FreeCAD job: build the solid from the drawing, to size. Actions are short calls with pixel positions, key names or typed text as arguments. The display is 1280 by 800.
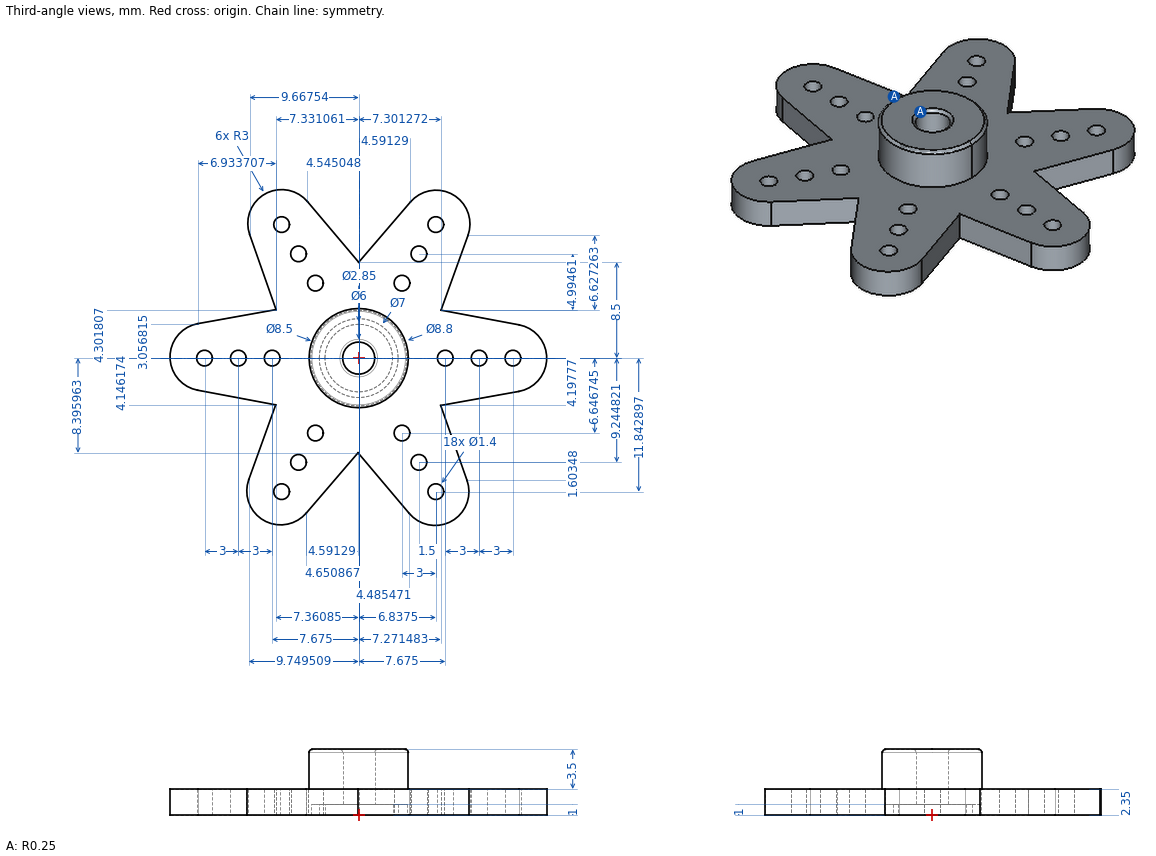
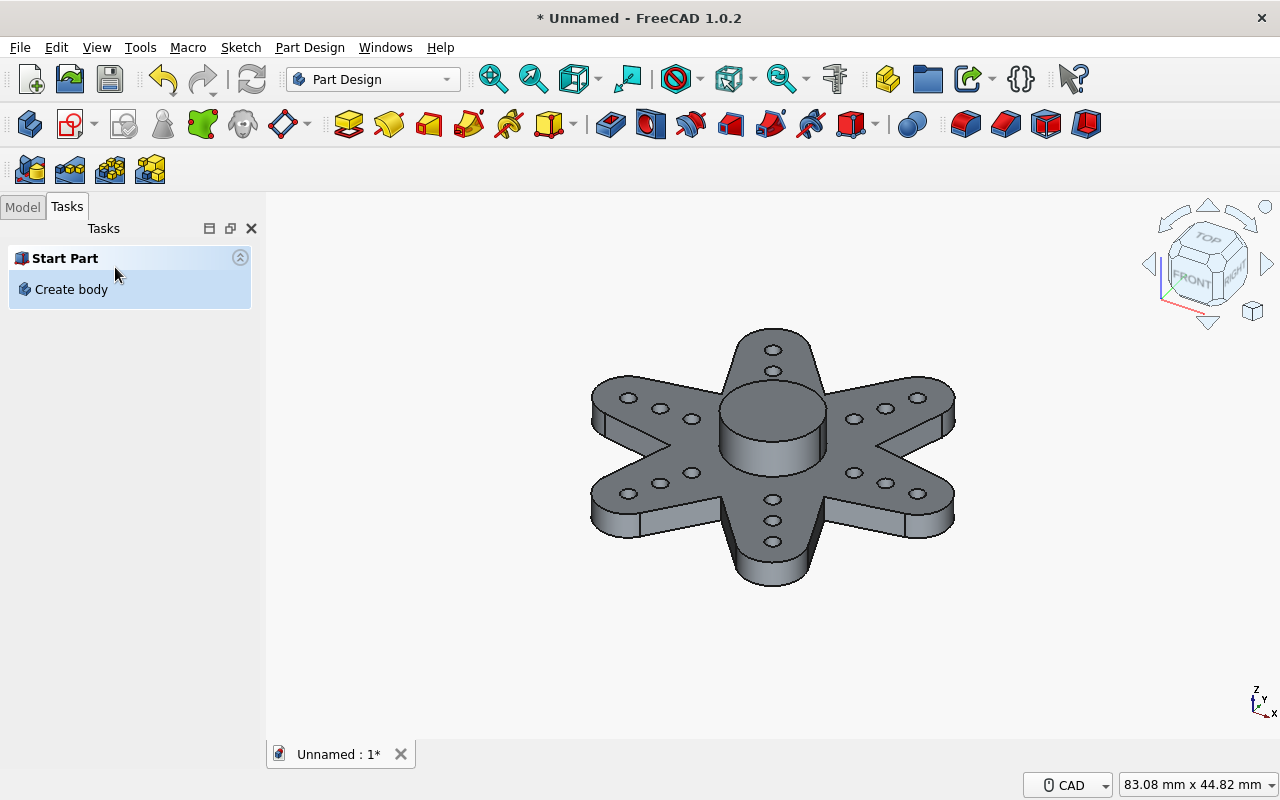
click(773, 410)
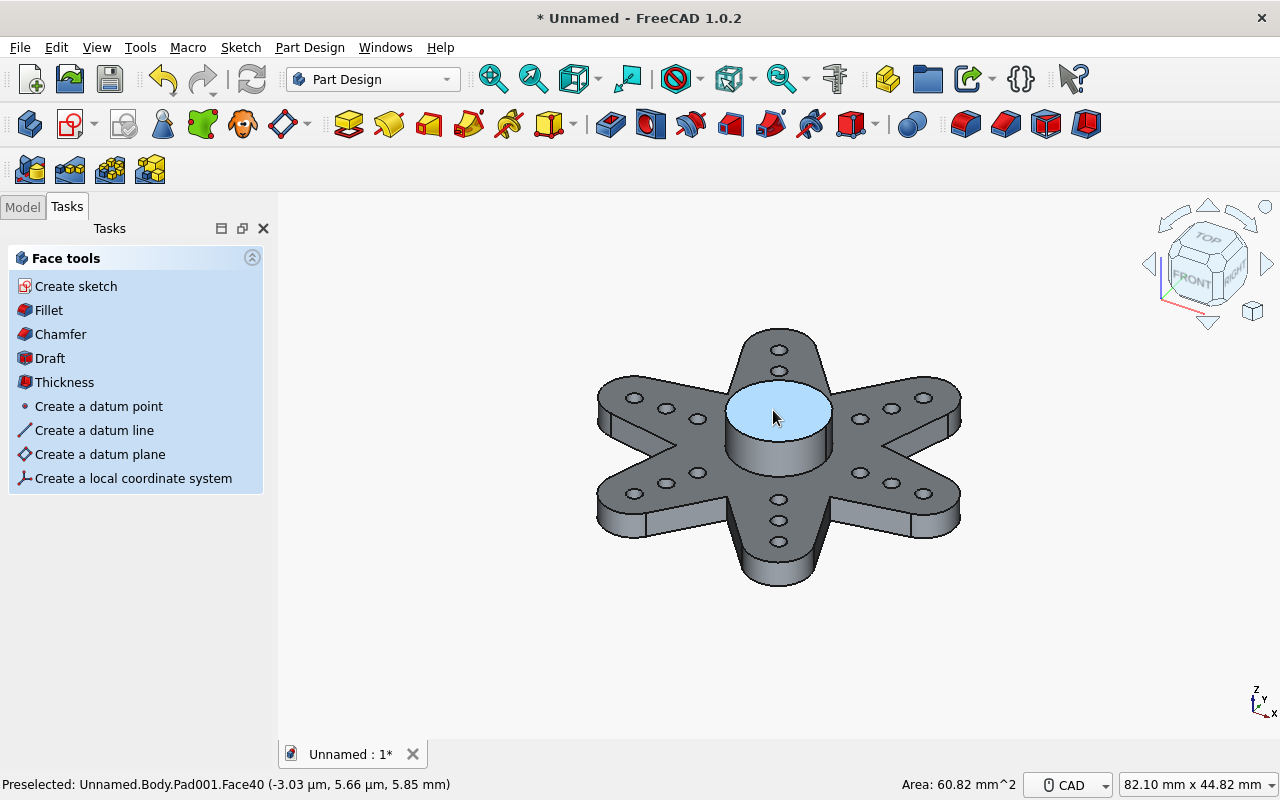
click(70, 124)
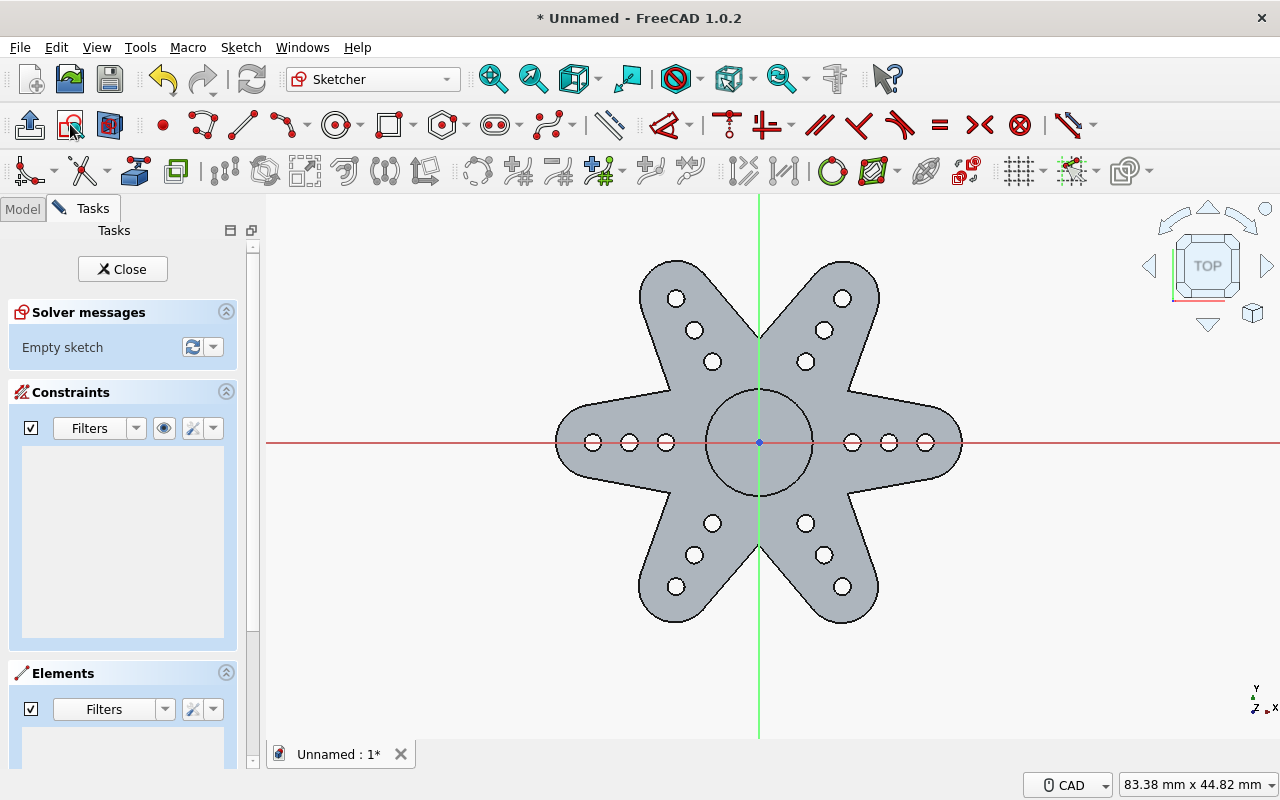
scroll(766, 440, up, 11)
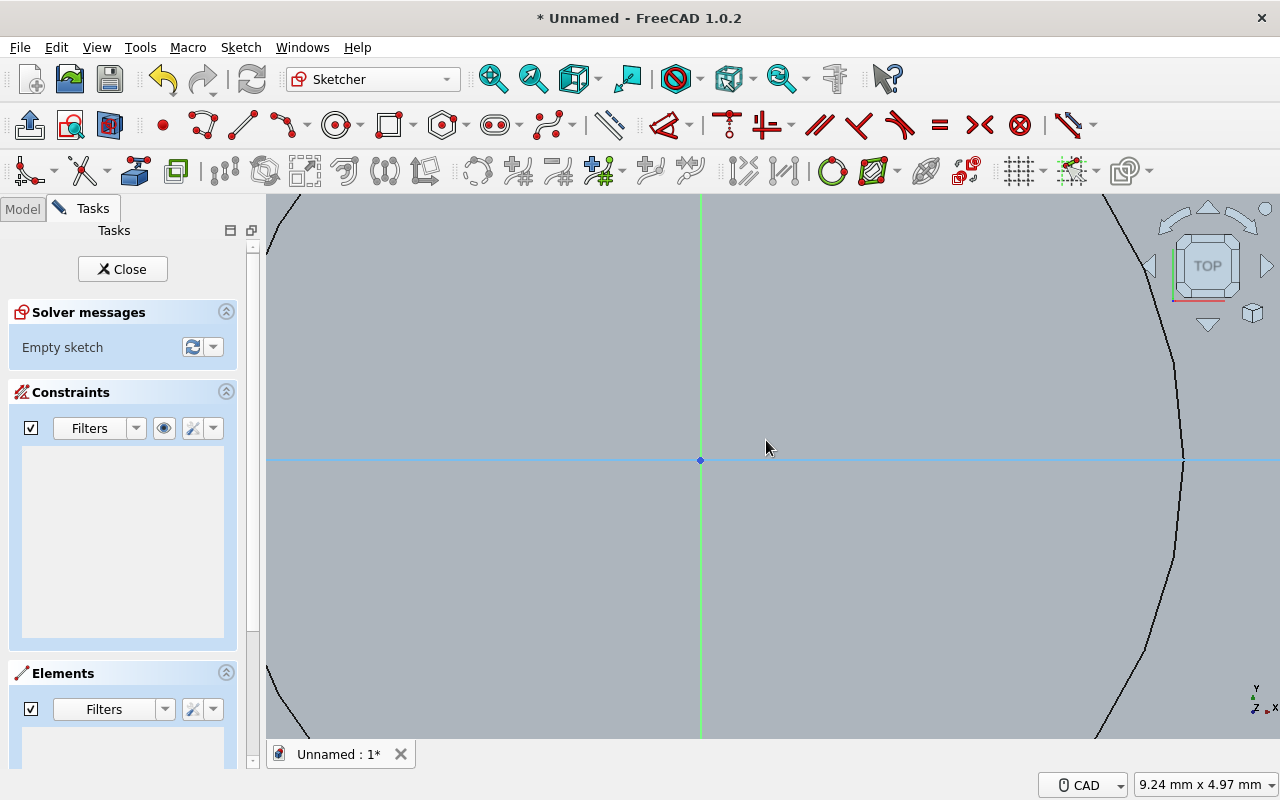
click(336, 126)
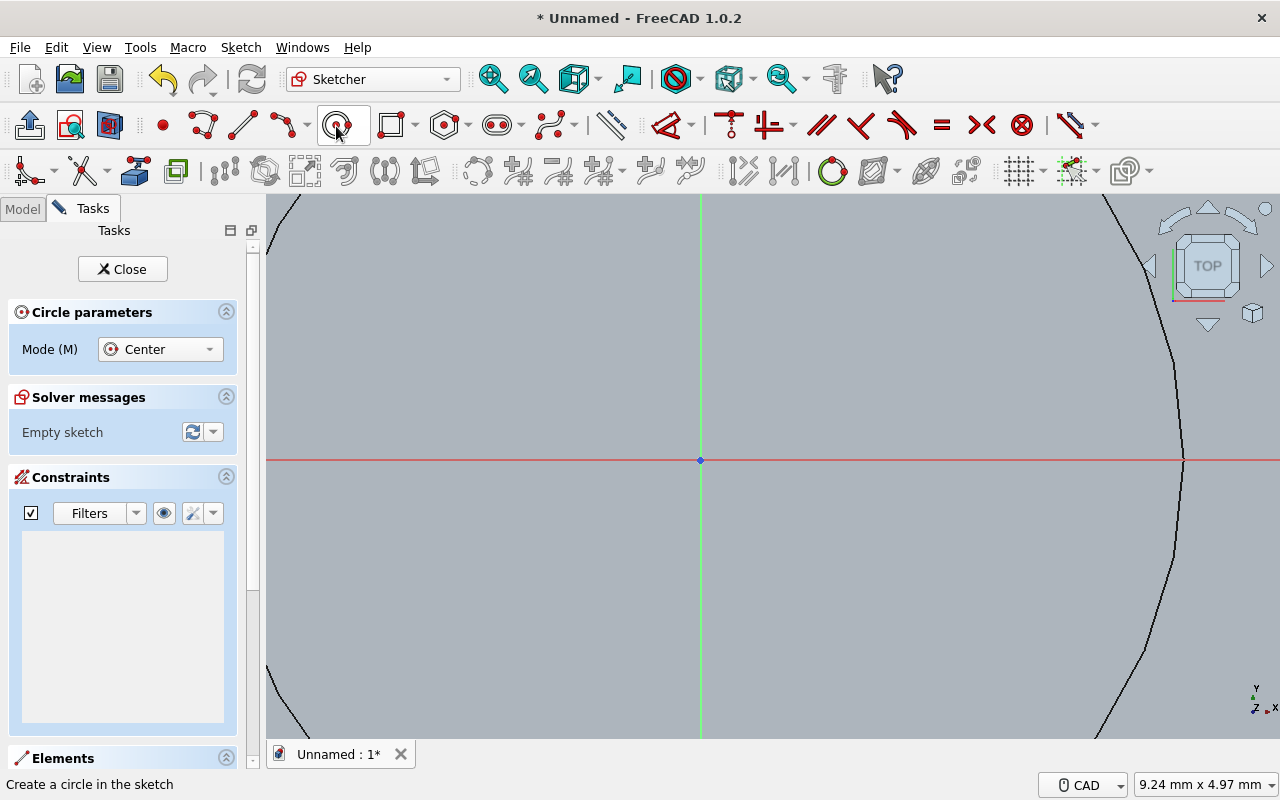
click(701, 460)
click(811, 349)
key(Escape)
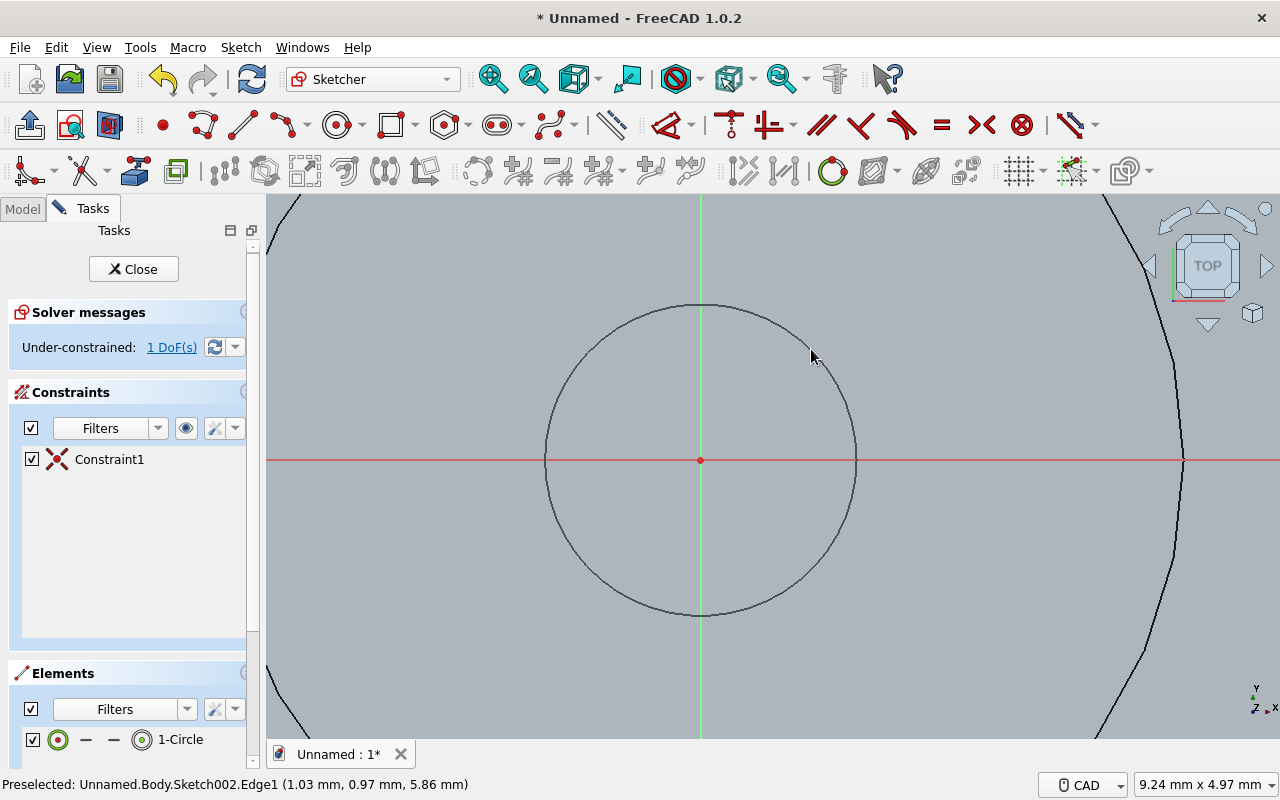
click(666, 126)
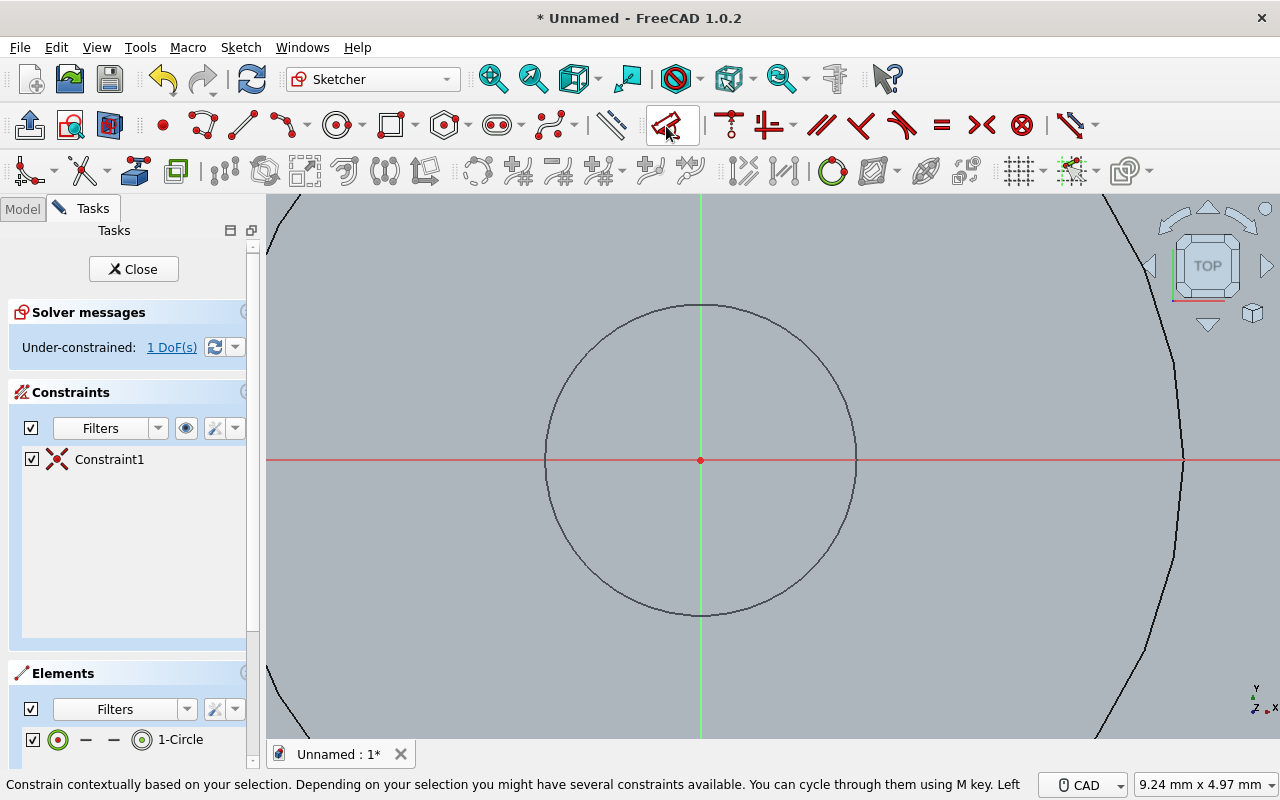
click(811, 350)
click(834, 327)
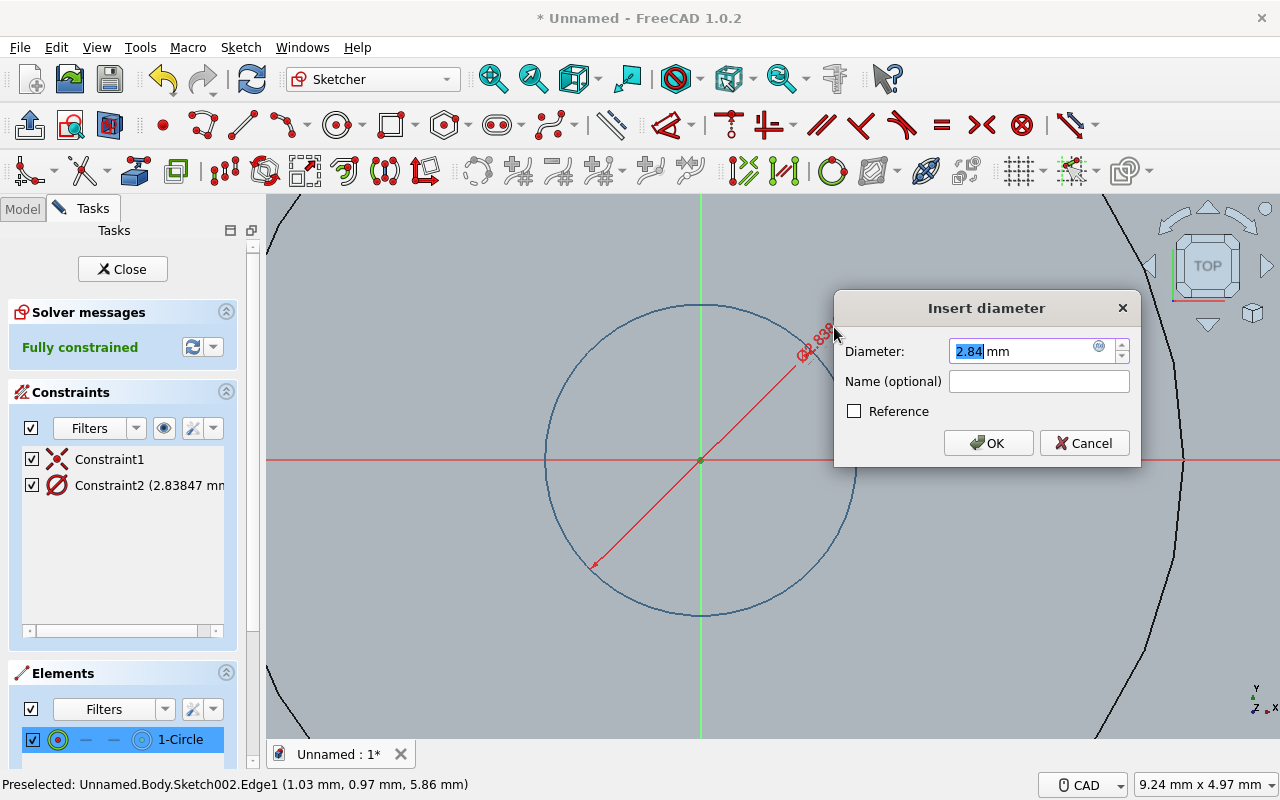
text(2.85)
key(Return)
key(Escape)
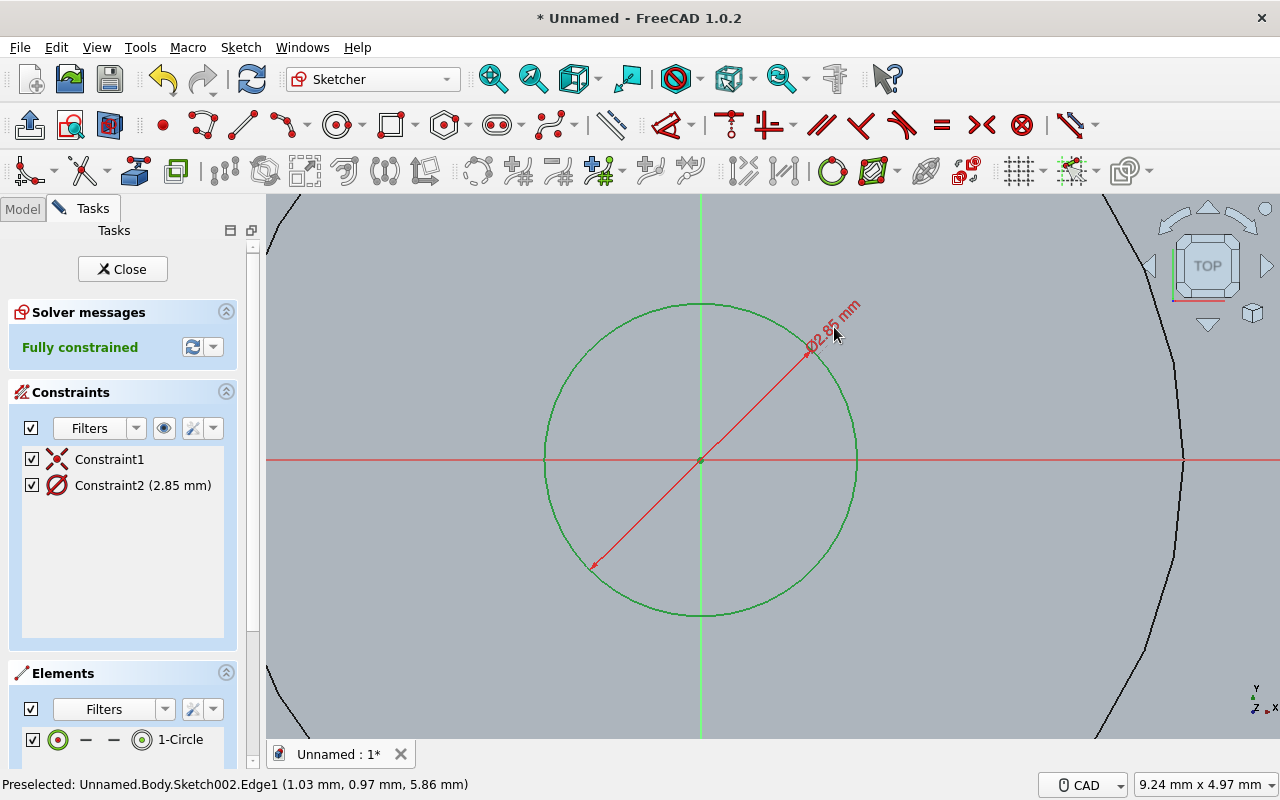
click(123, 269)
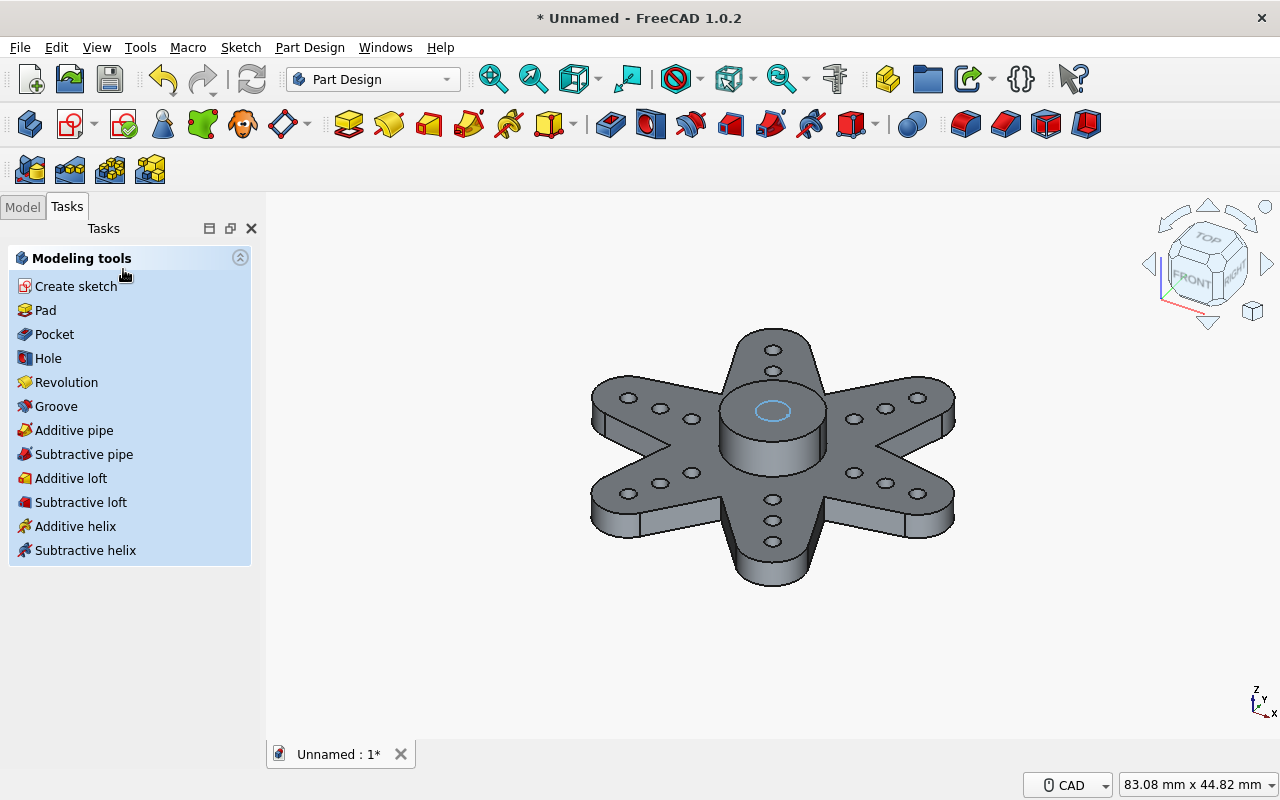
click(612, 124)